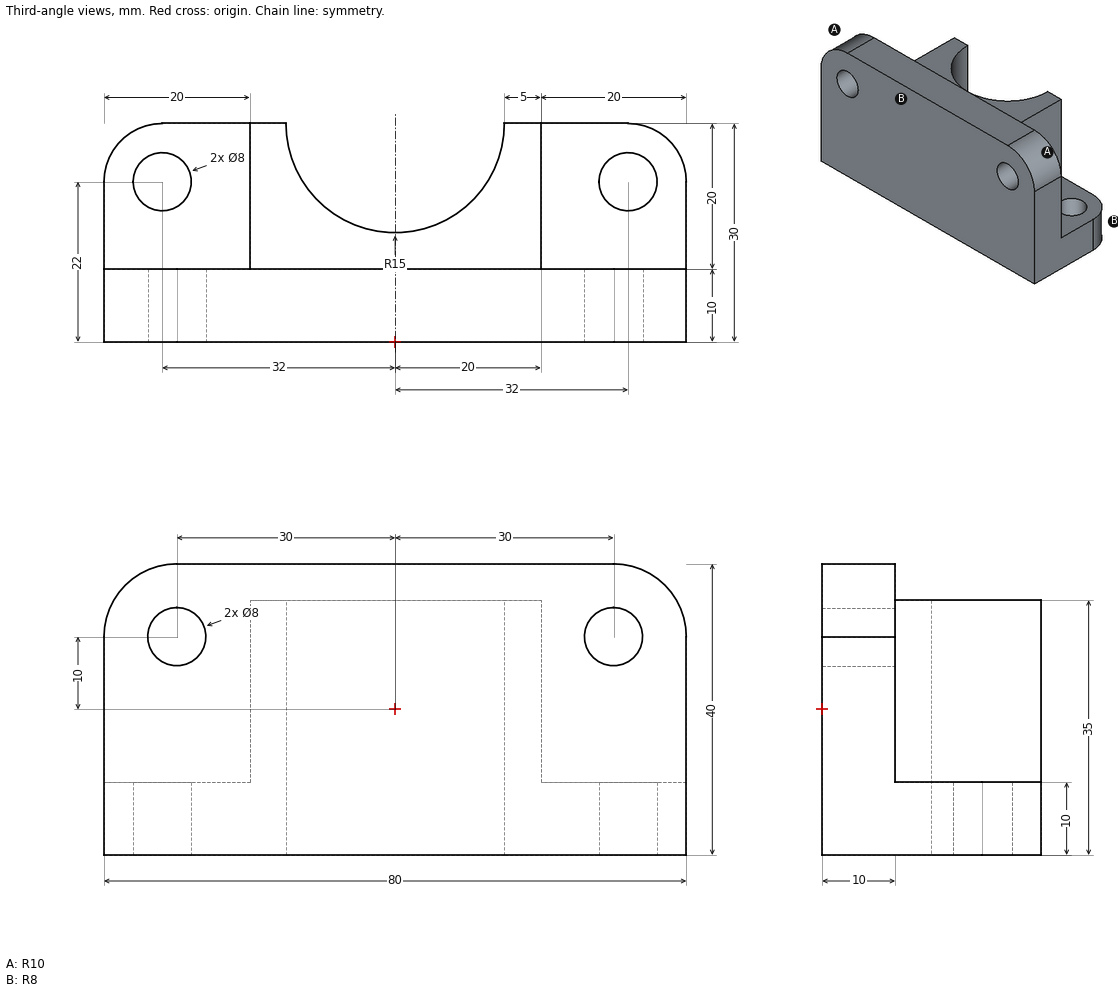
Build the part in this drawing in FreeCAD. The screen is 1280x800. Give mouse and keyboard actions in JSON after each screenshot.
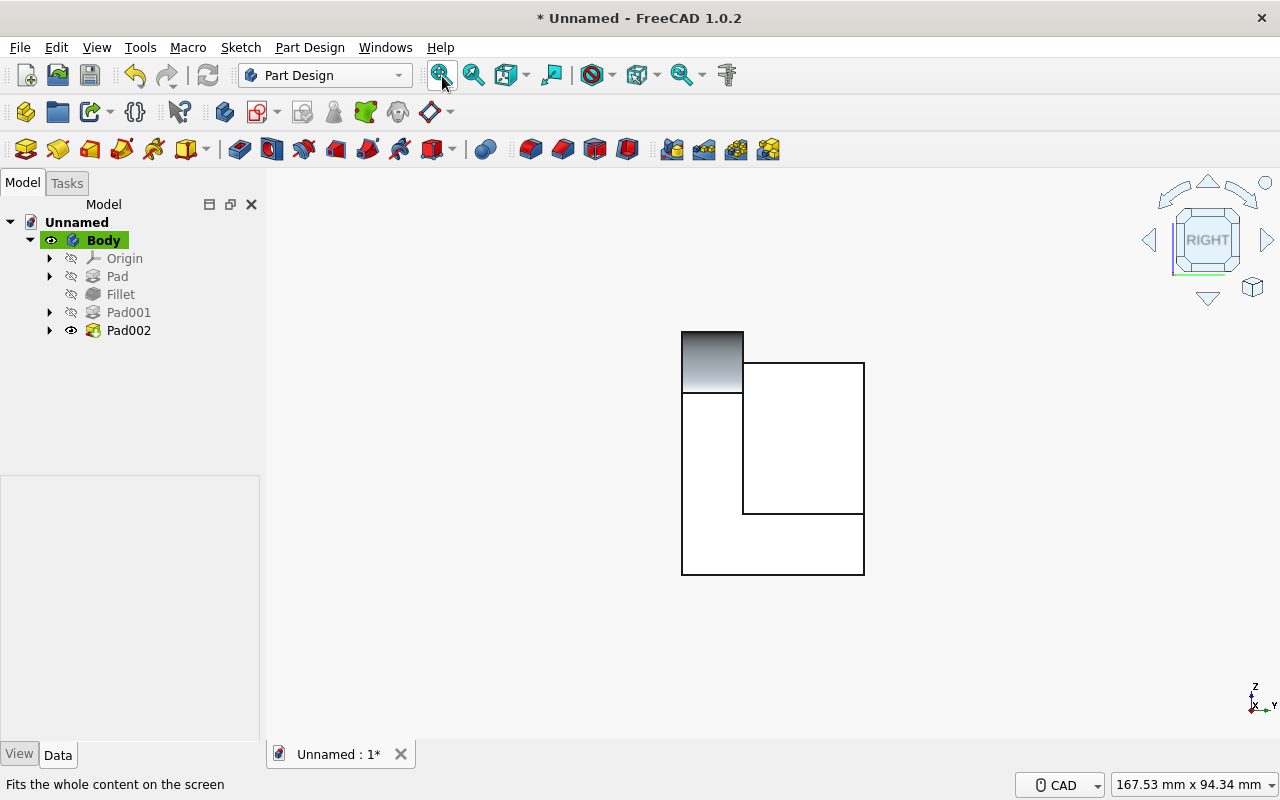
{"action": "left_click", "coordinate": [864, 543]}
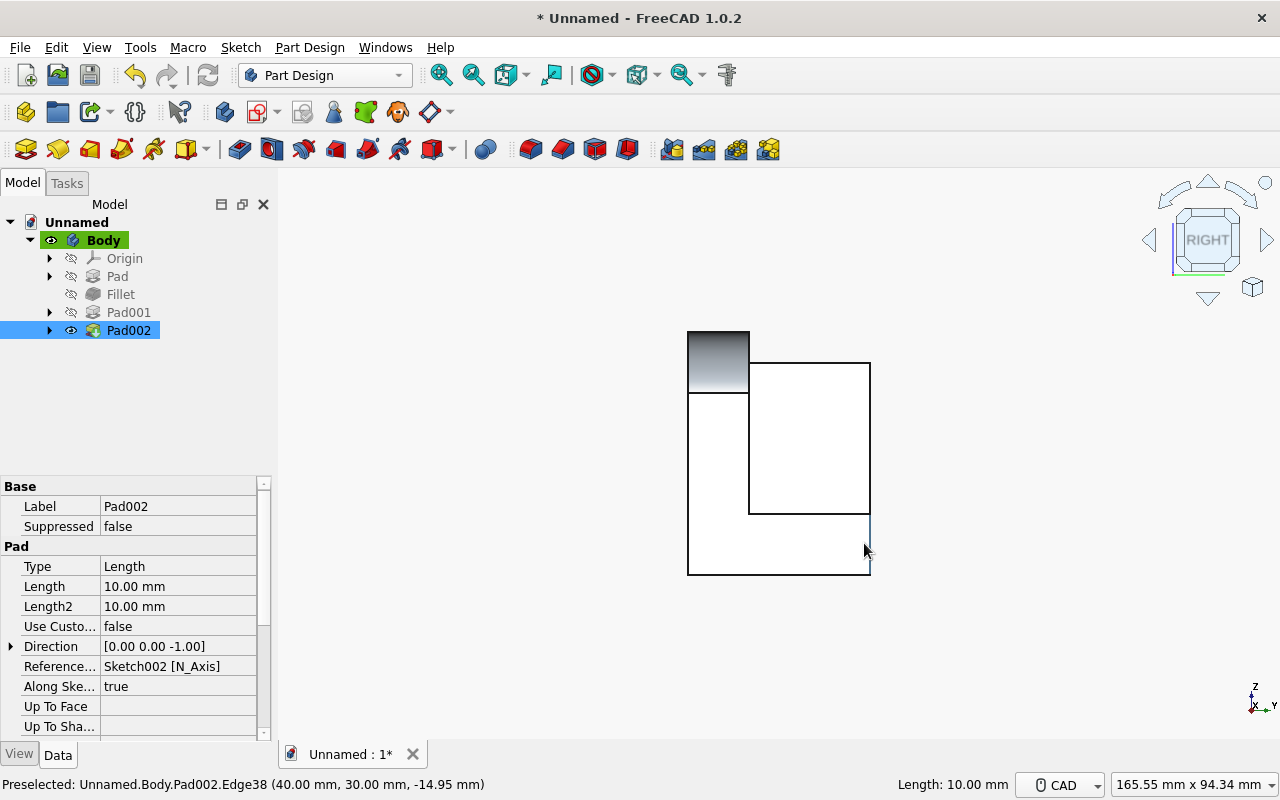
{"action": "key", "text": "5"}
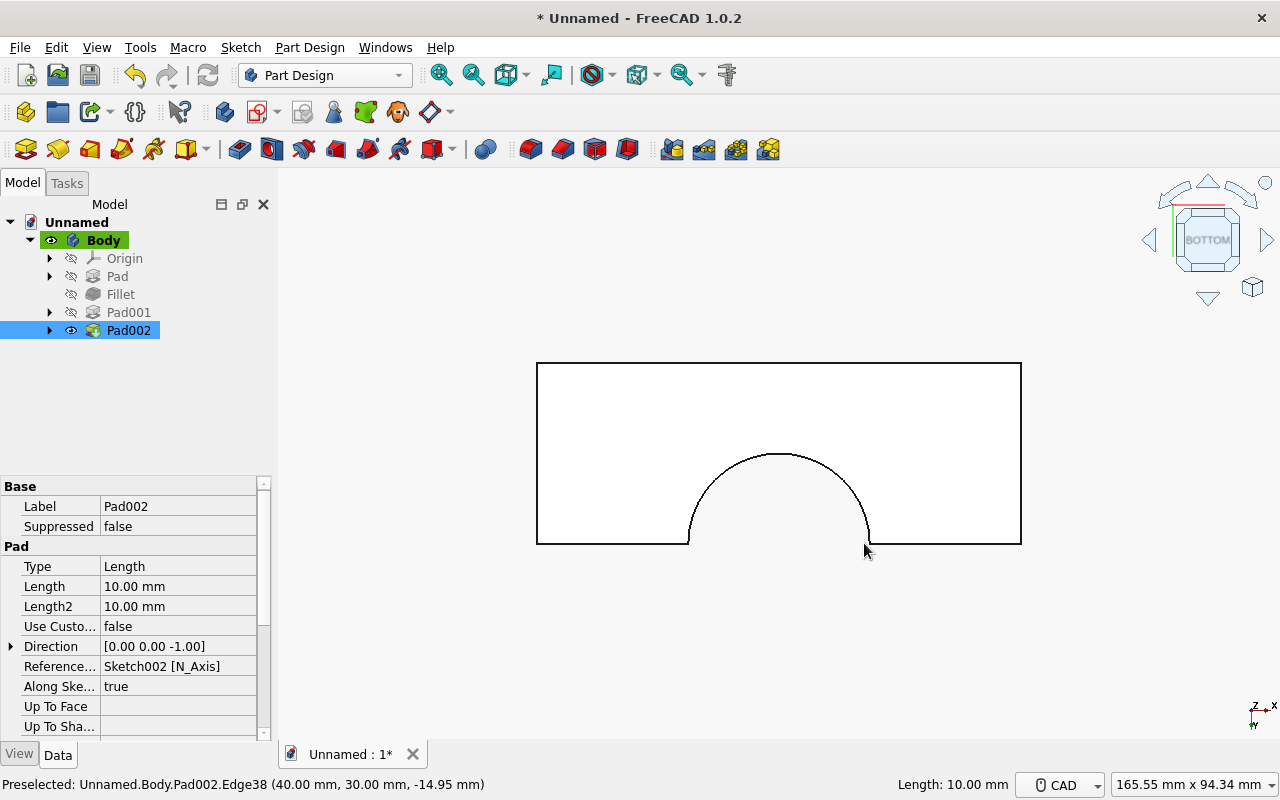
{"action": "key", "text": "4"}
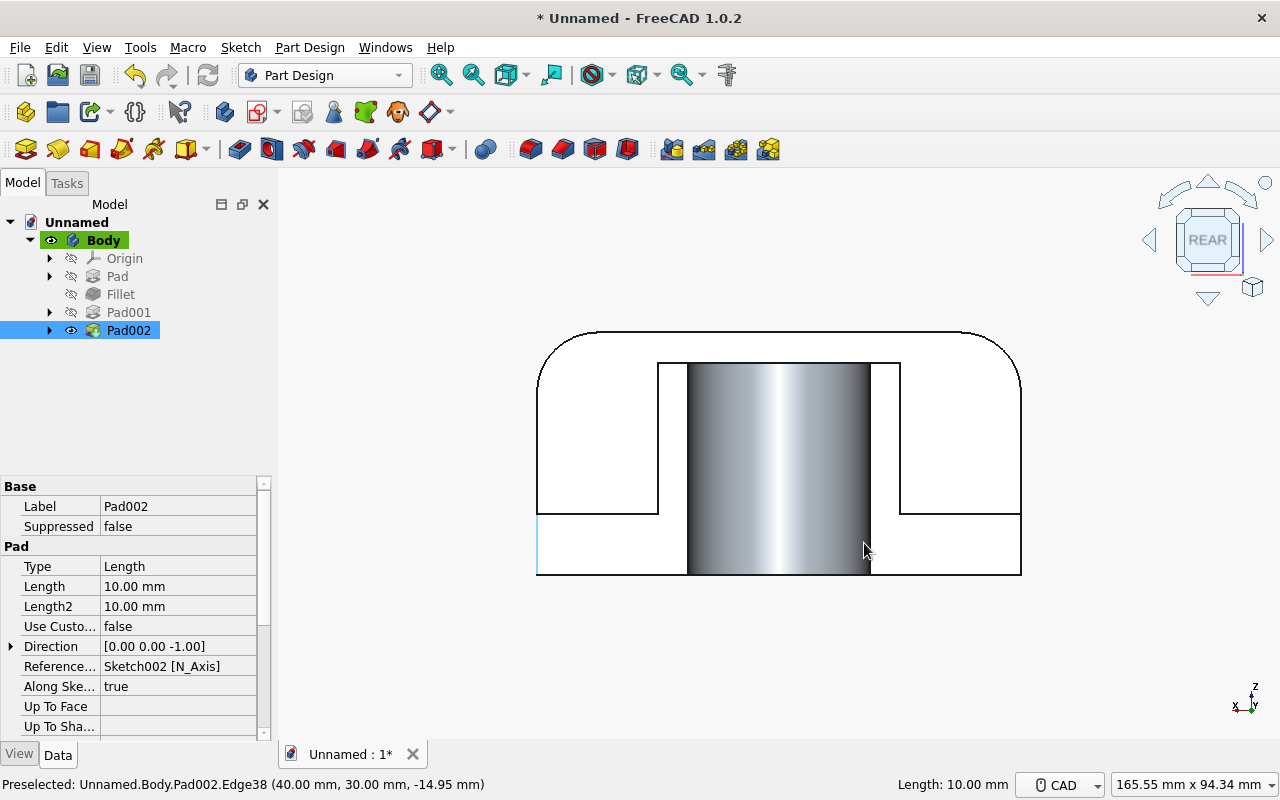
{"action": "left_click", "coordinate": [1021, 543], "text": "ctrl"}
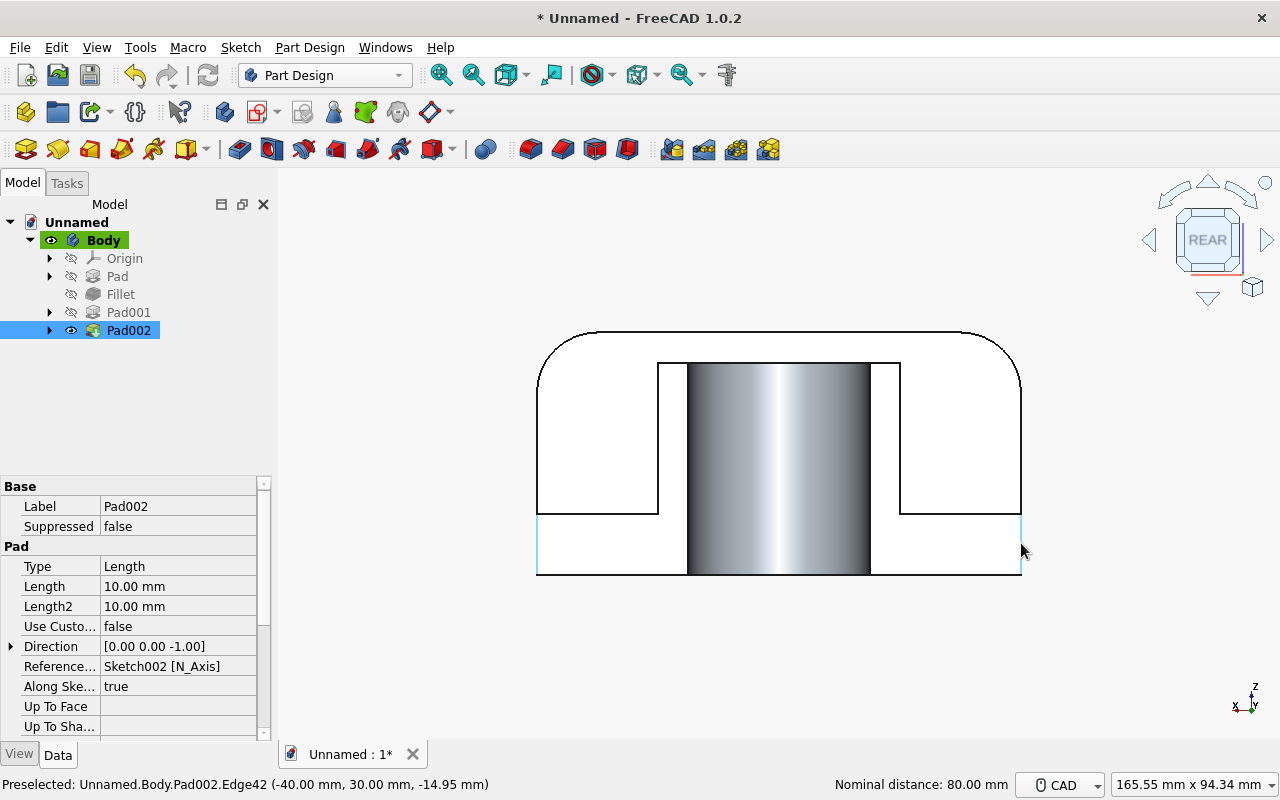
{"action": "left_click", "coordinate": [532, 150]}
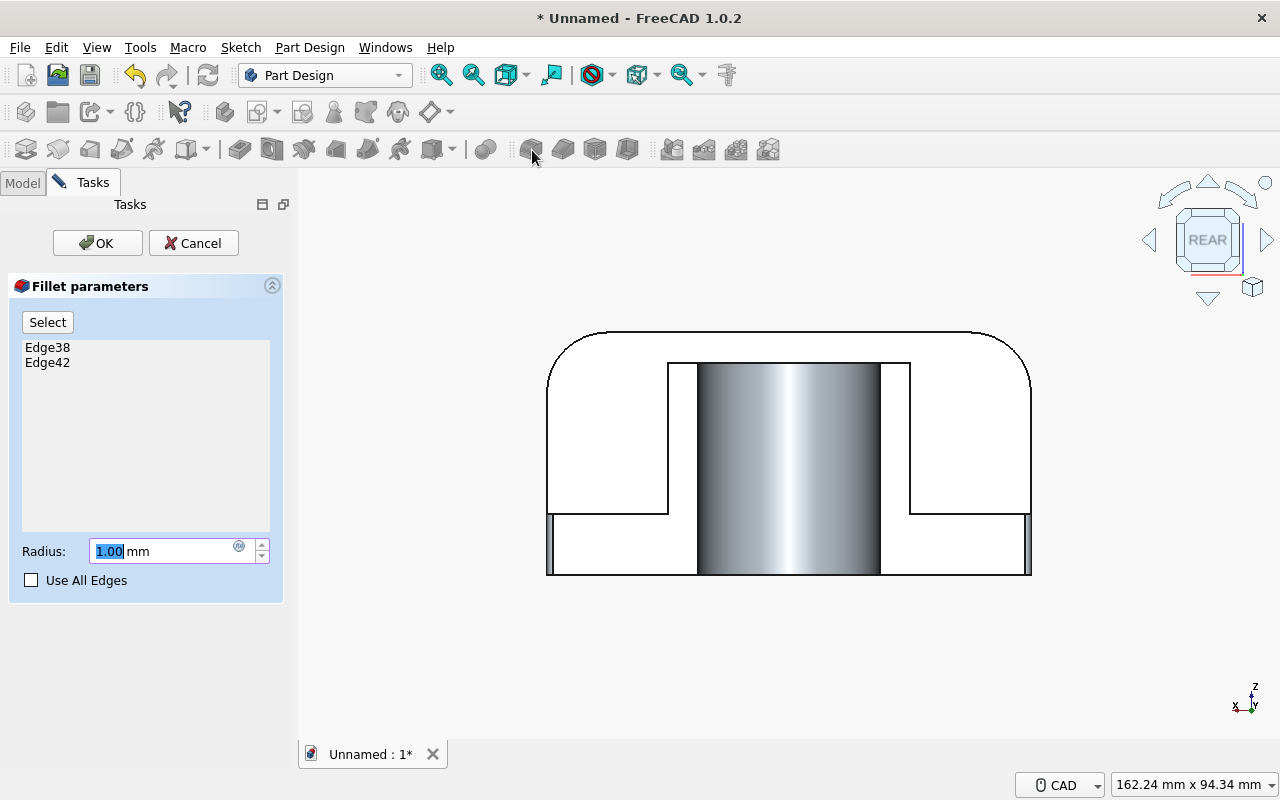
{"action": "type", "text": "8"}
{"action": "key", "text": "Tab"}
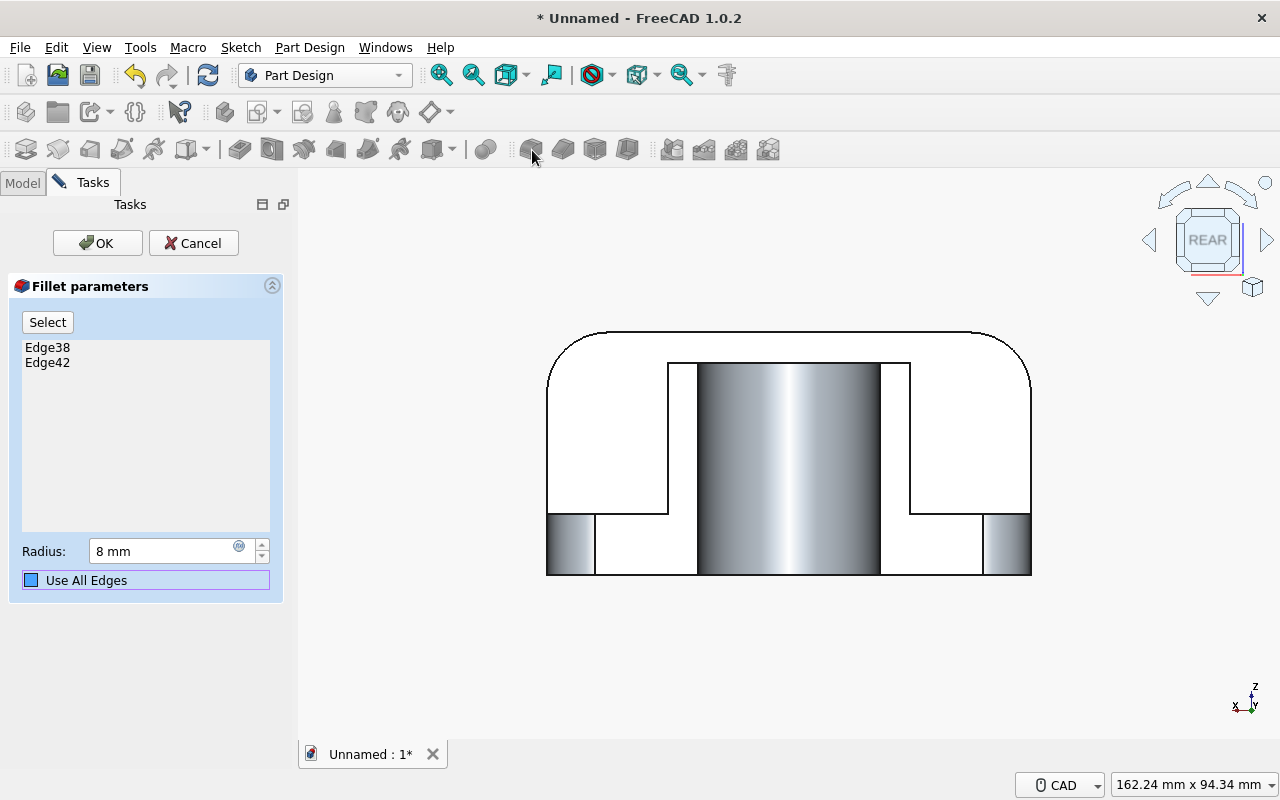
{"action": "left_click", "coordinate": [98, 243]}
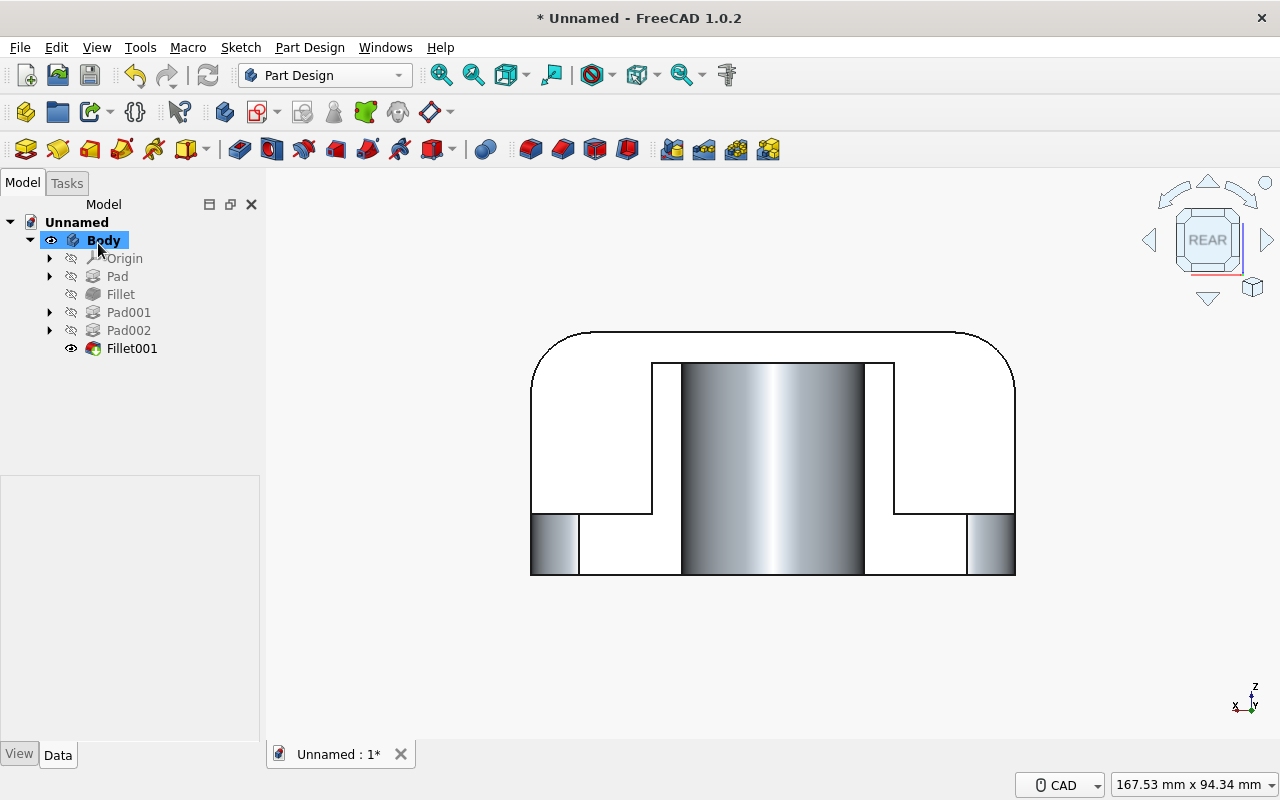
{"action": "key", "text": "5"}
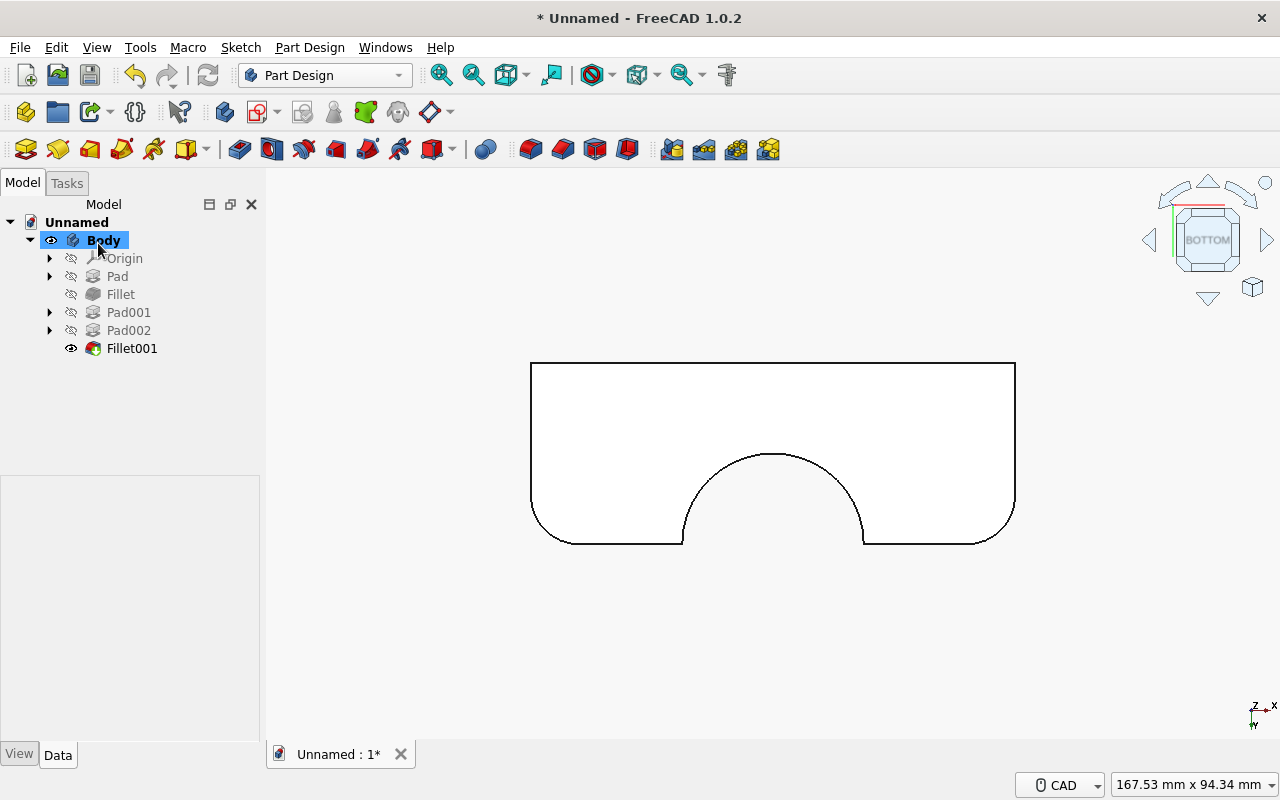
{"action": "left_click", "coordinate": [911, 452]}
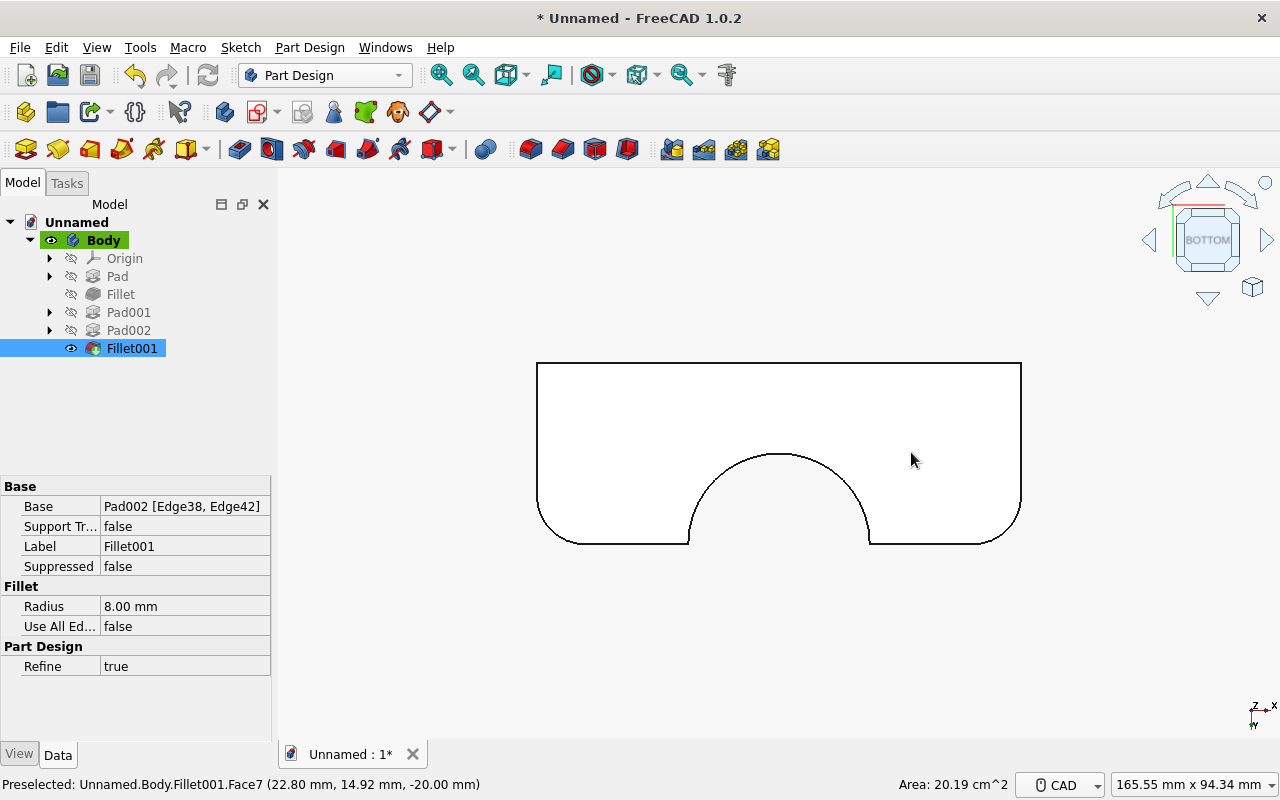
{"action": "left_click", "coordinate": [258, 112]}